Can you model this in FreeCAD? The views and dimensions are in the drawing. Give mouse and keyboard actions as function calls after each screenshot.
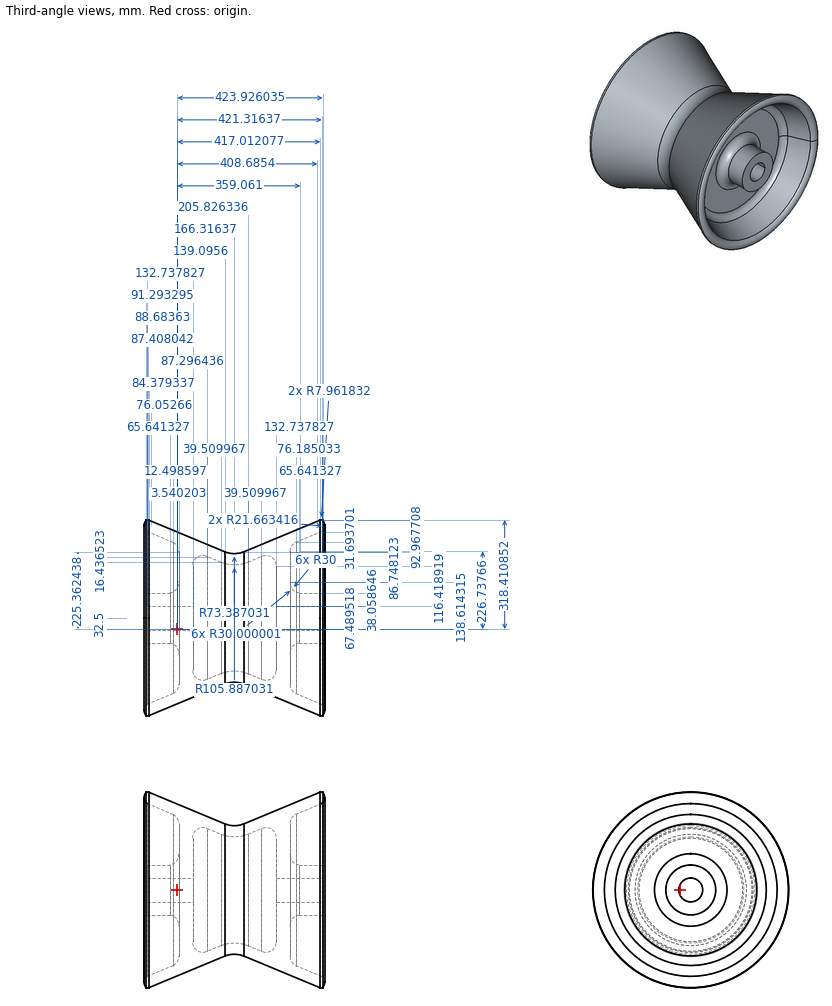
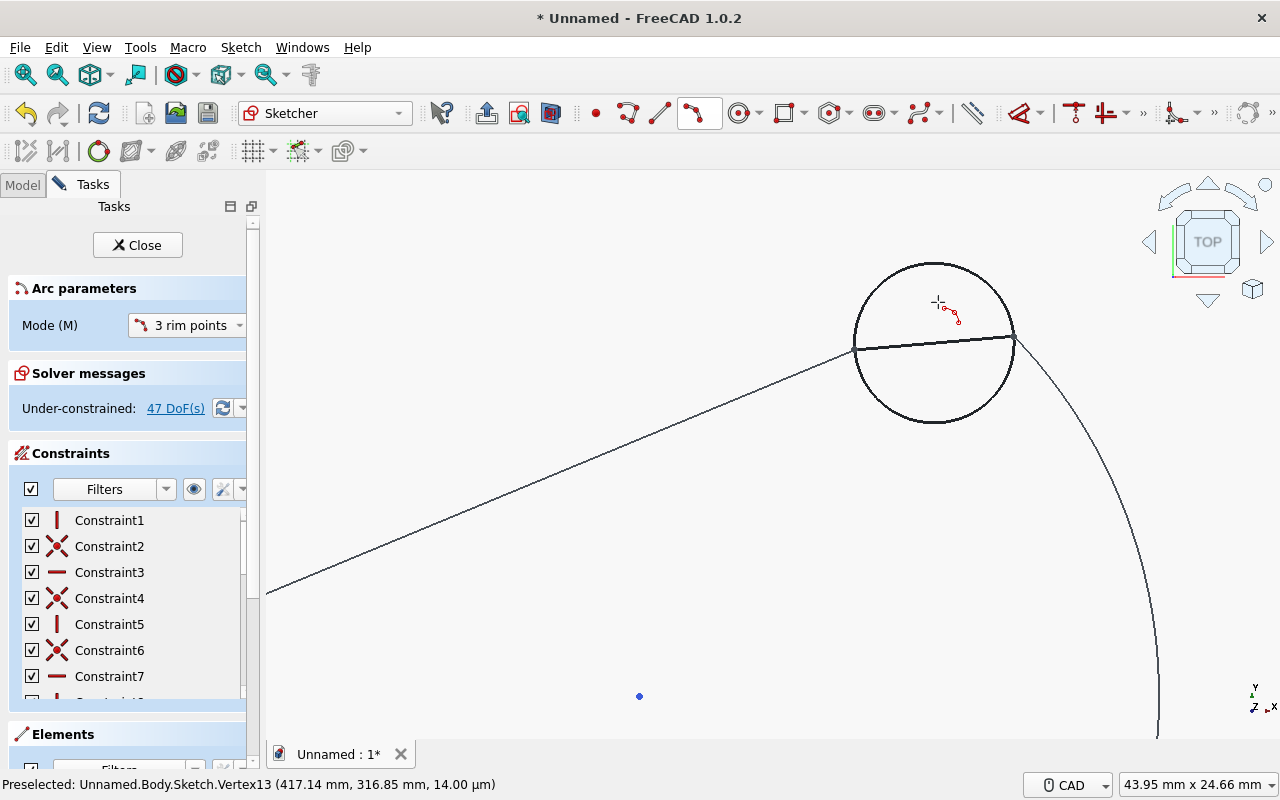
click(933, 300)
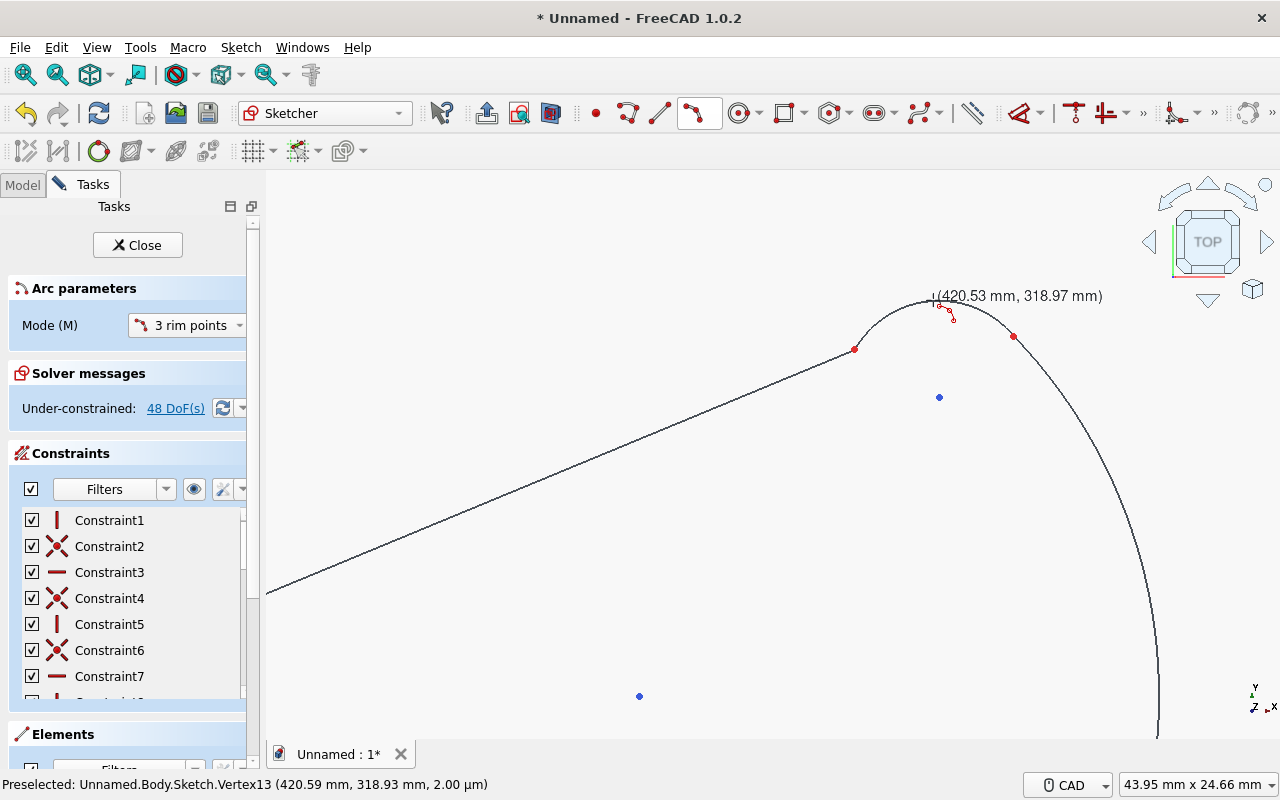
scroll(1000, 270, down, 15)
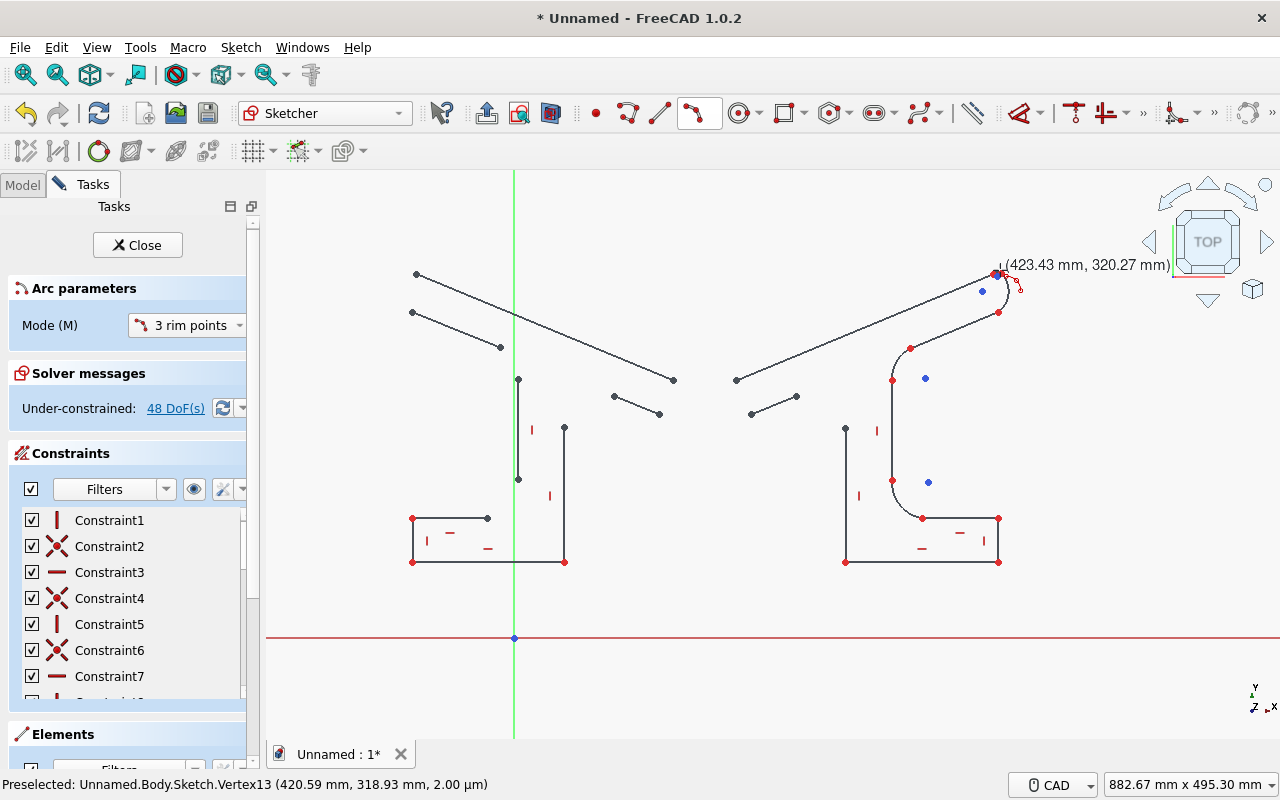
click(737, 380)
click(673, 380)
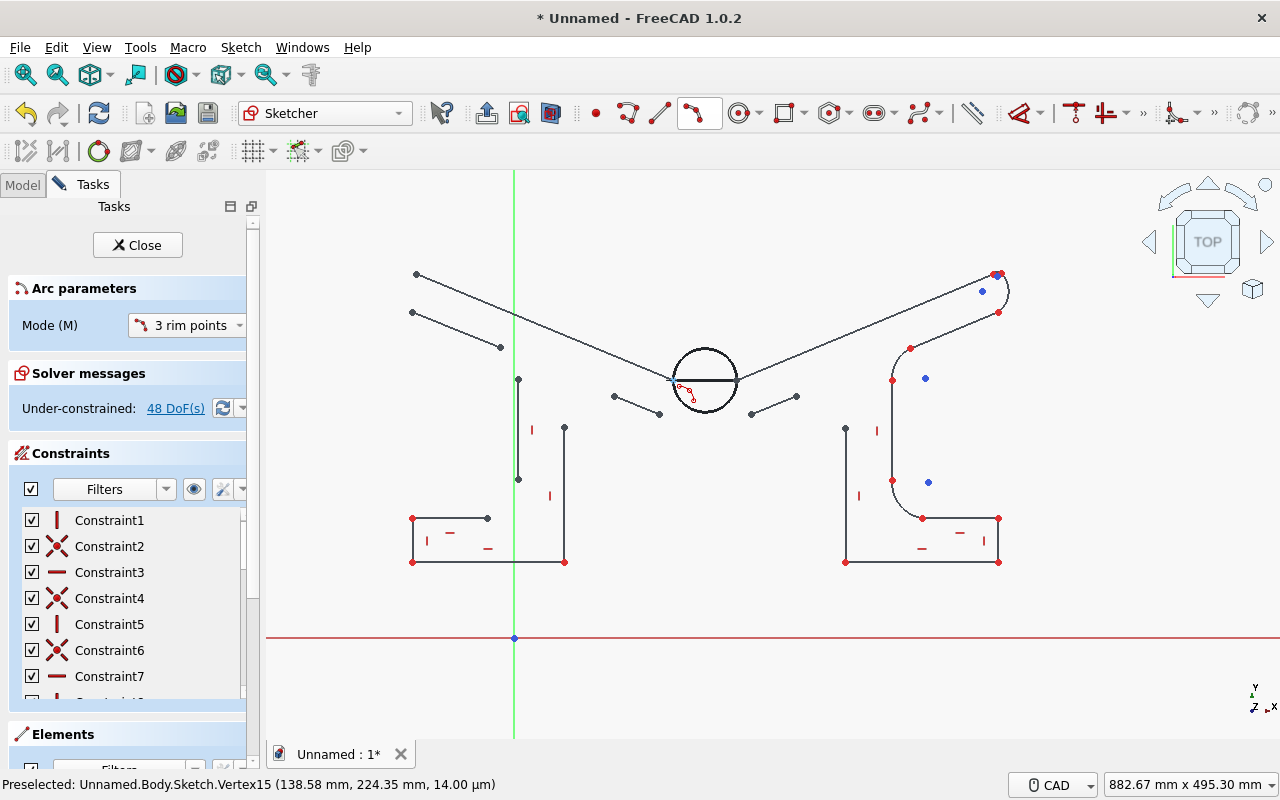
scroll(705, 385, up, 5)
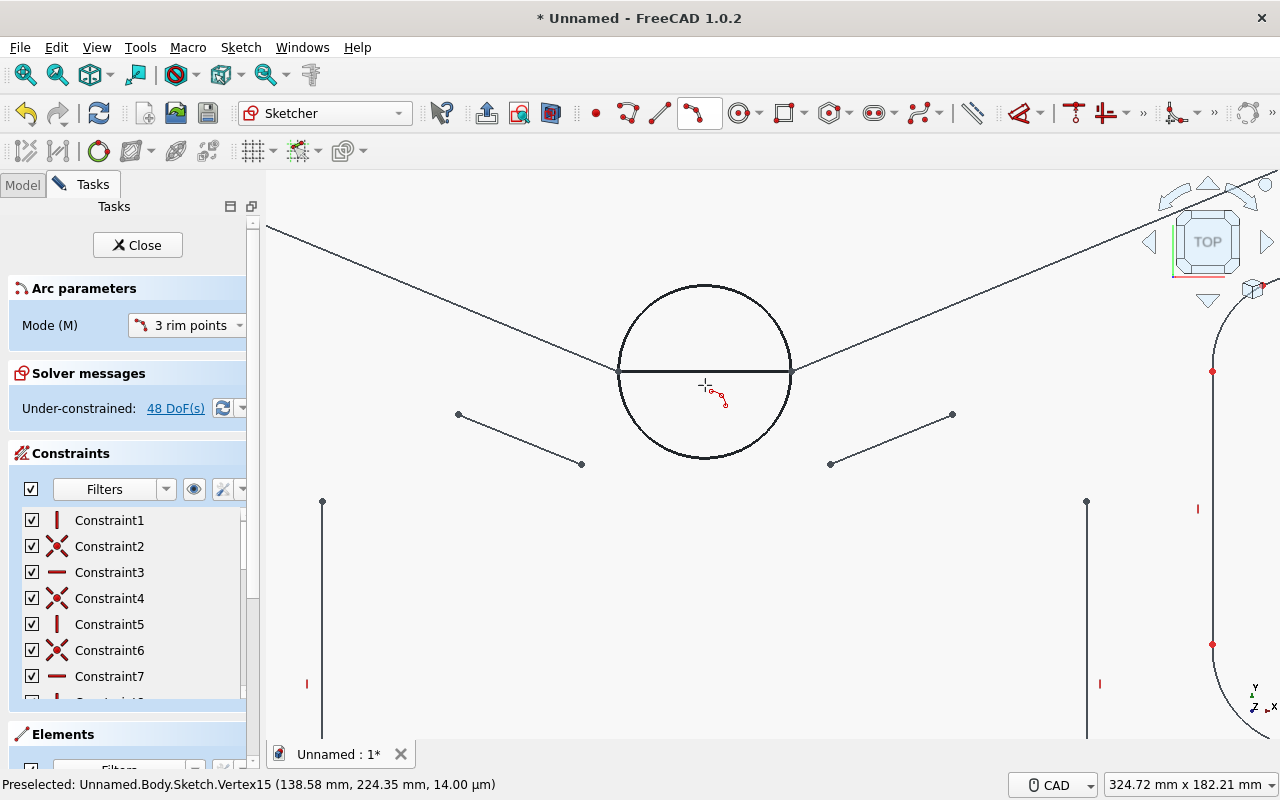
click(705, 385)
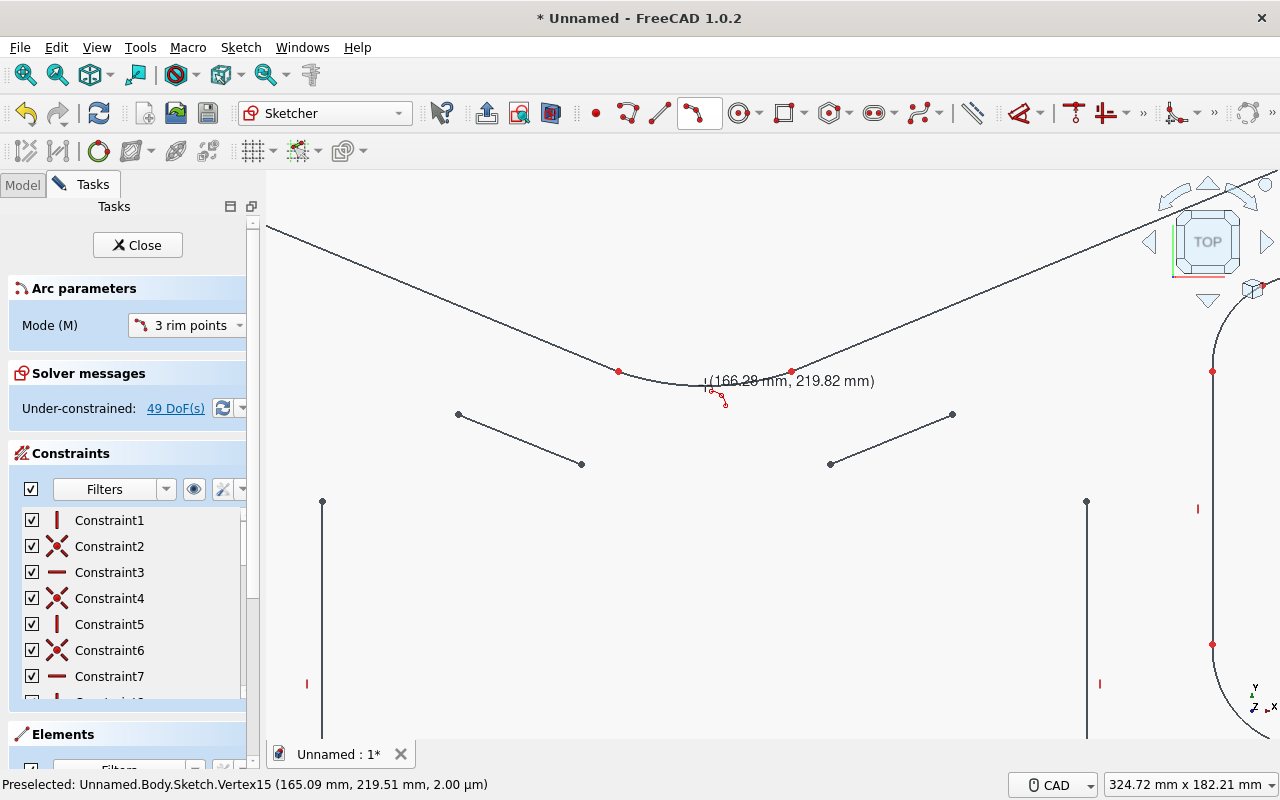
scroll(704, 403, down, 6)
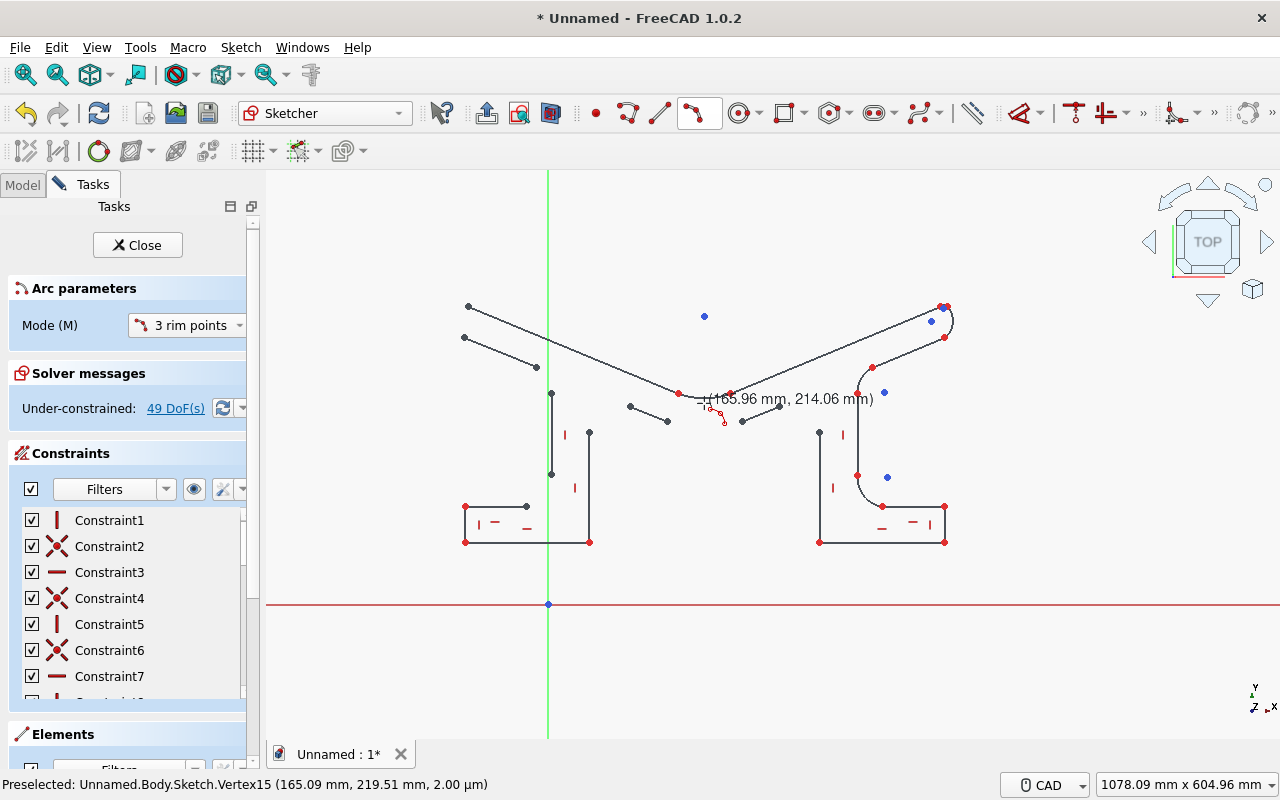
click(469, 307)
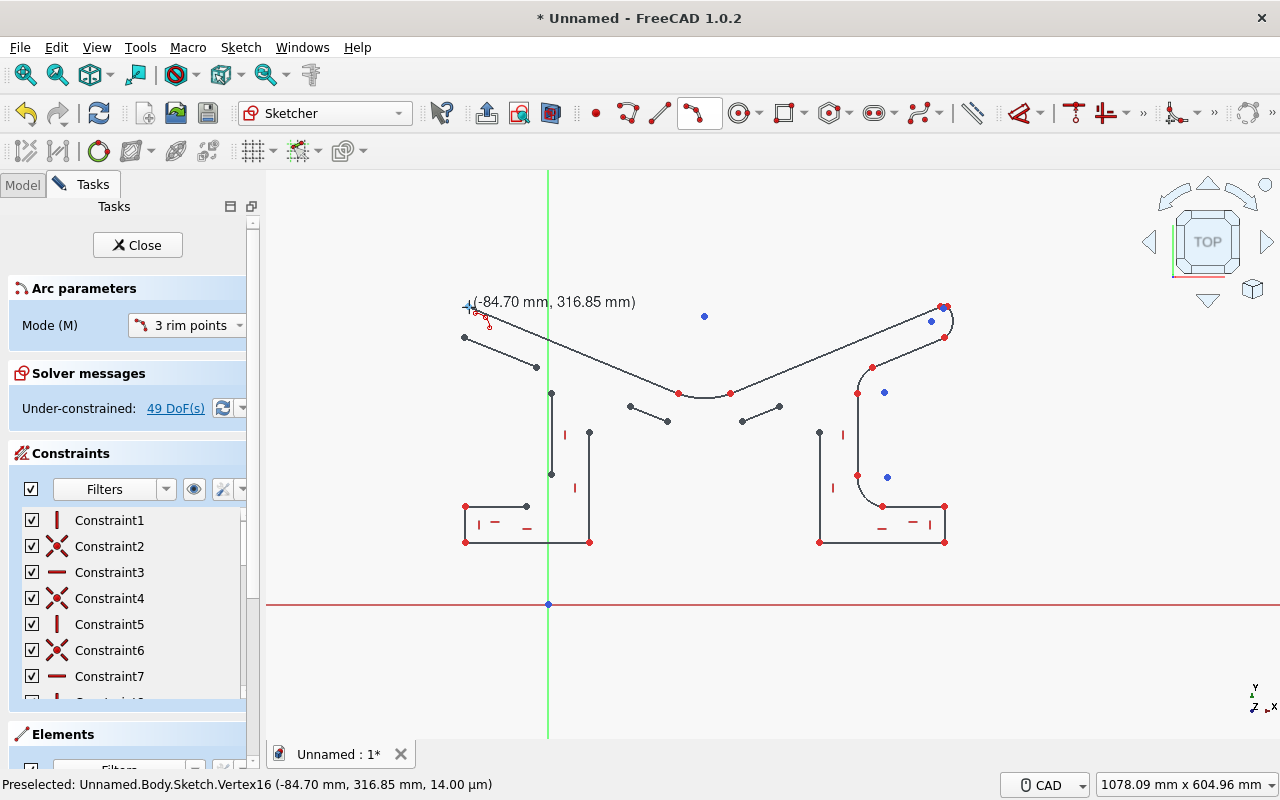
scroll(462, 306, up, 5)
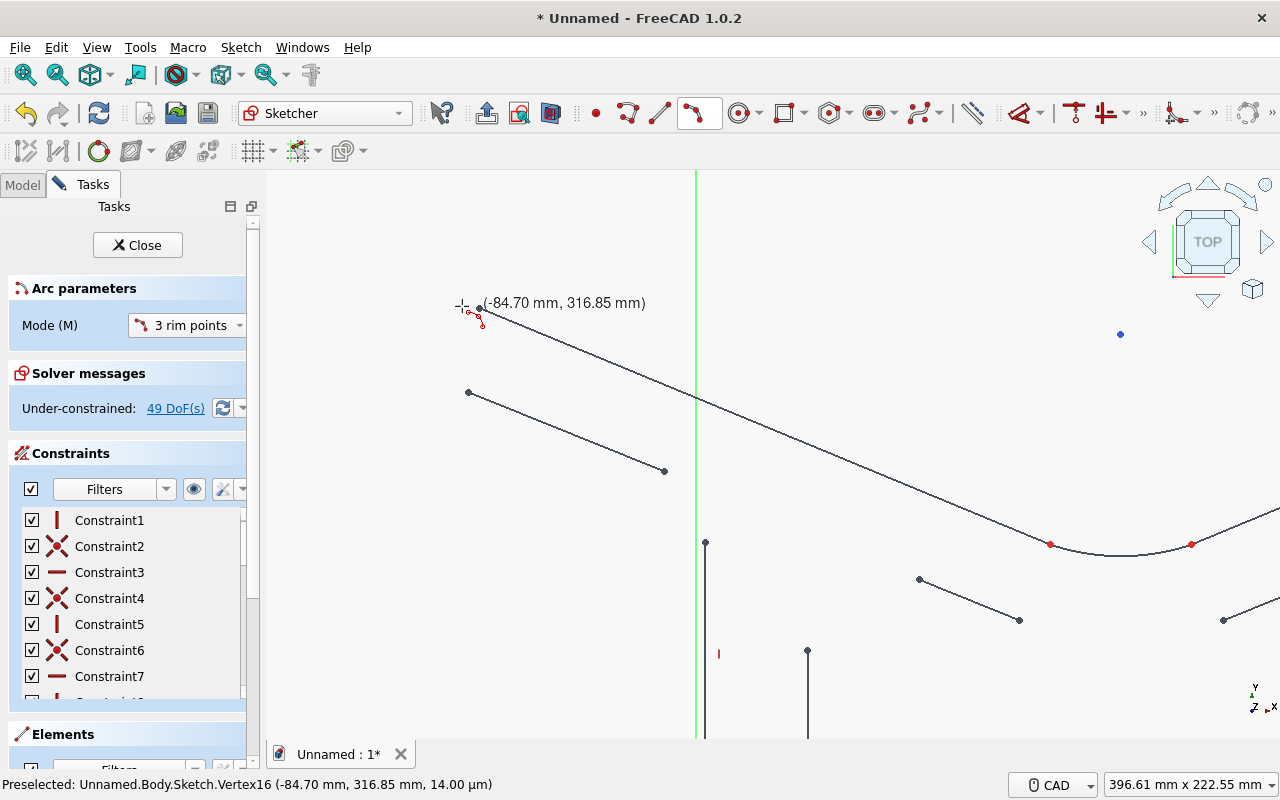
click(463, 305)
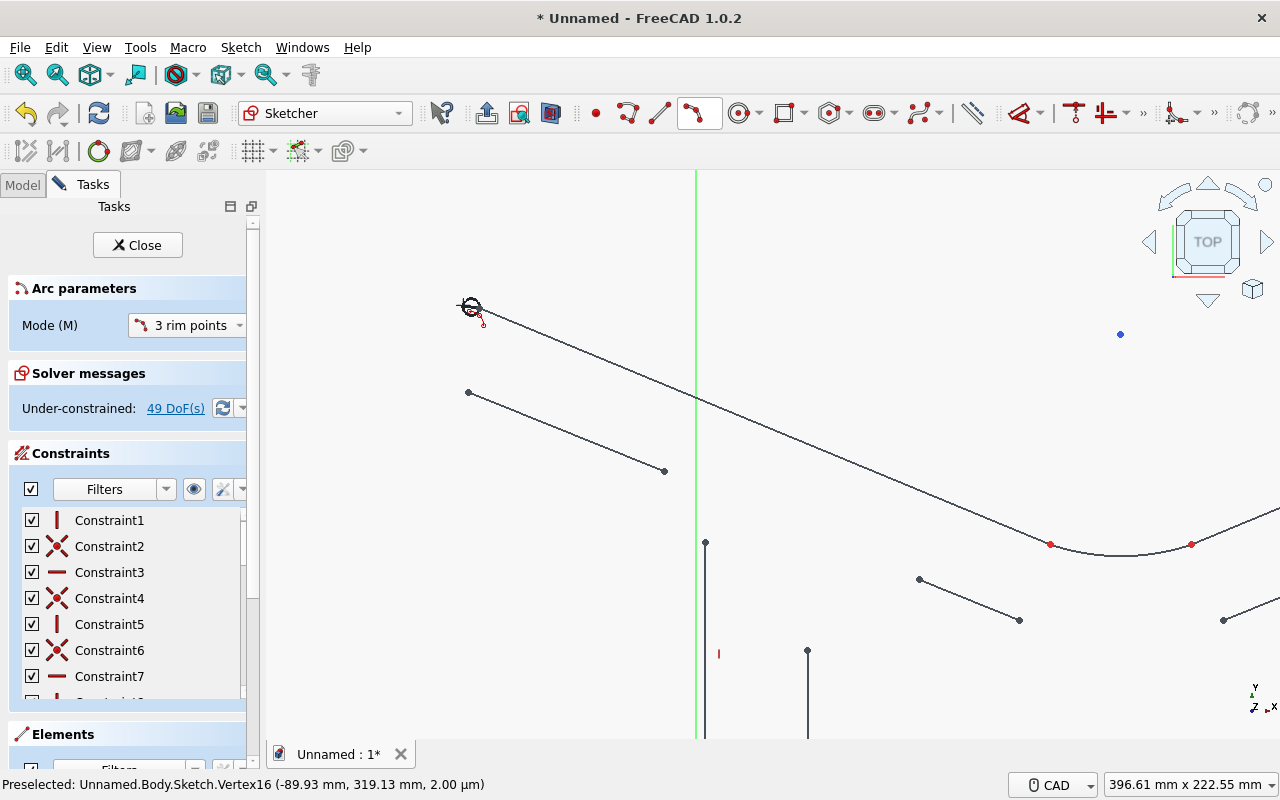
scroll(471, 303, up, 11)